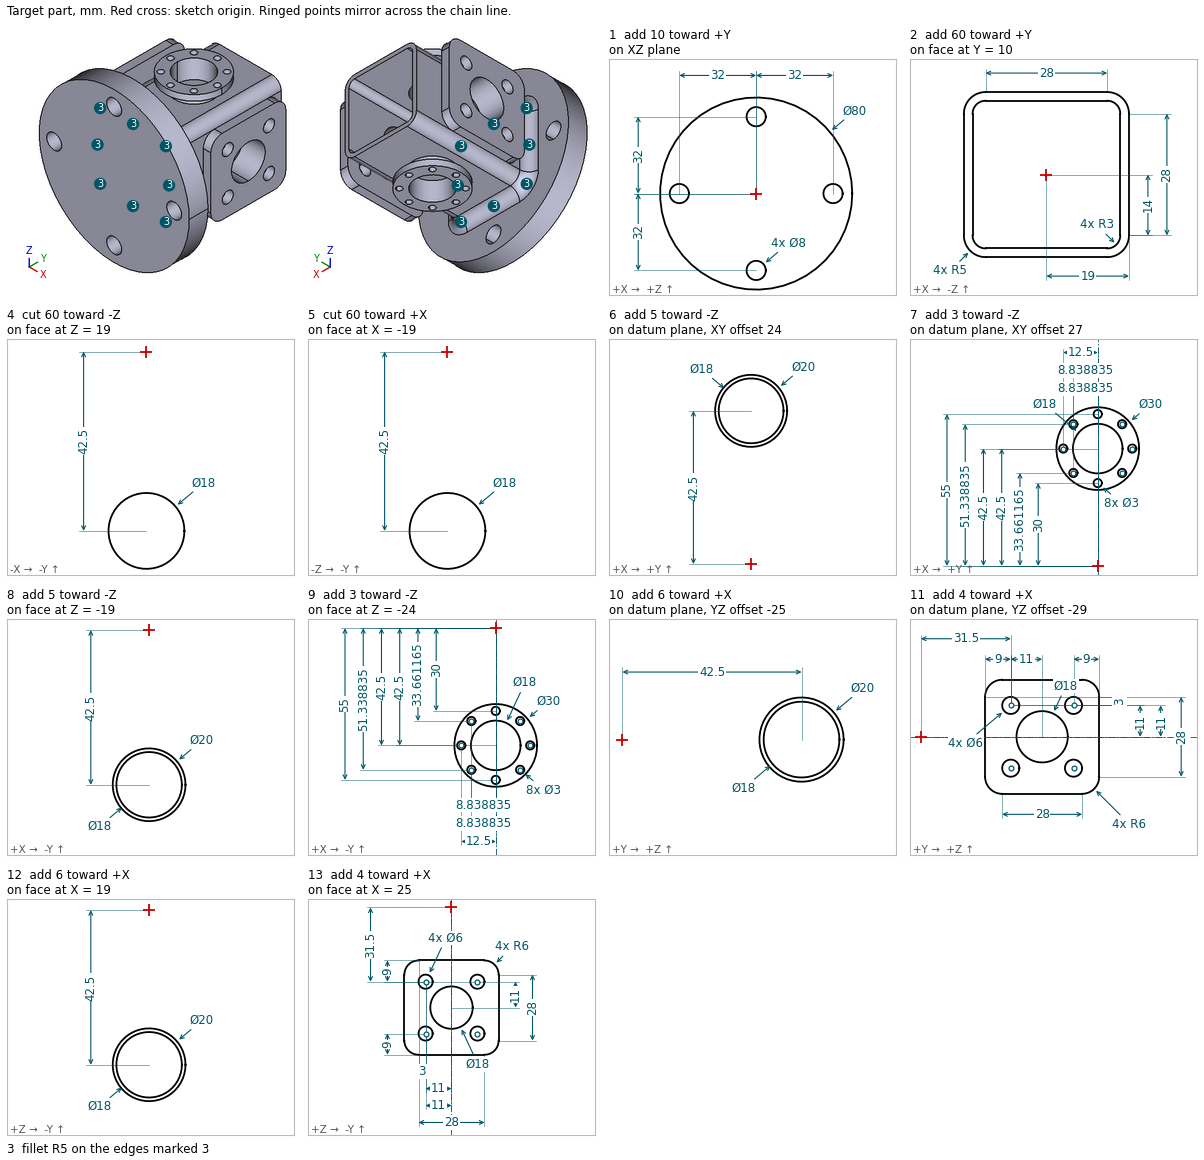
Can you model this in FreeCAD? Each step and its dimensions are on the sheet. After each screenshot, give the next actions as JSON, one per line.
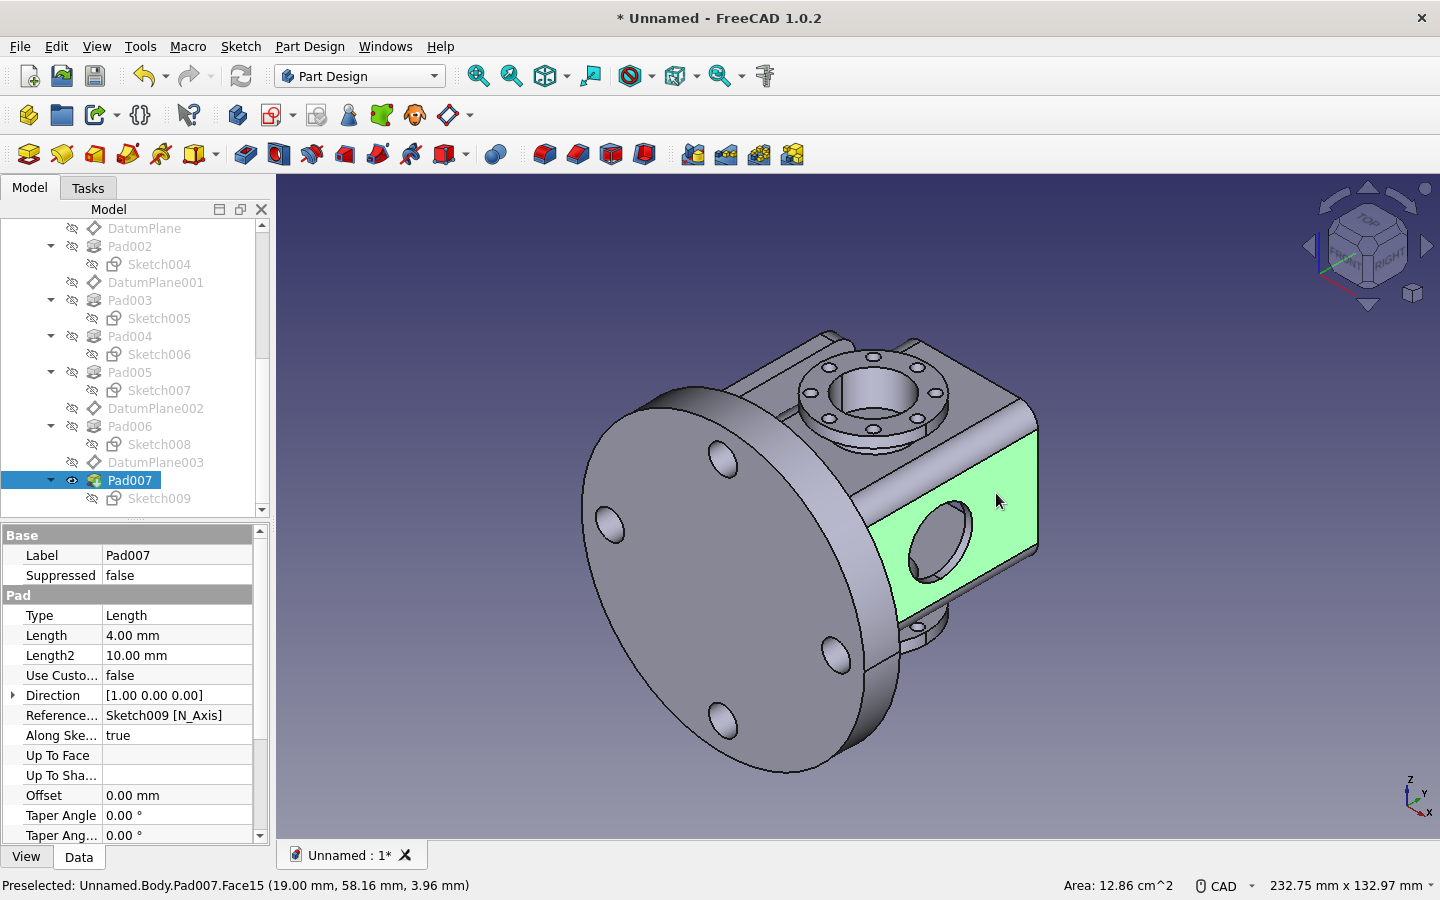
{"action": "left_click", "coordinate": [270, 116]}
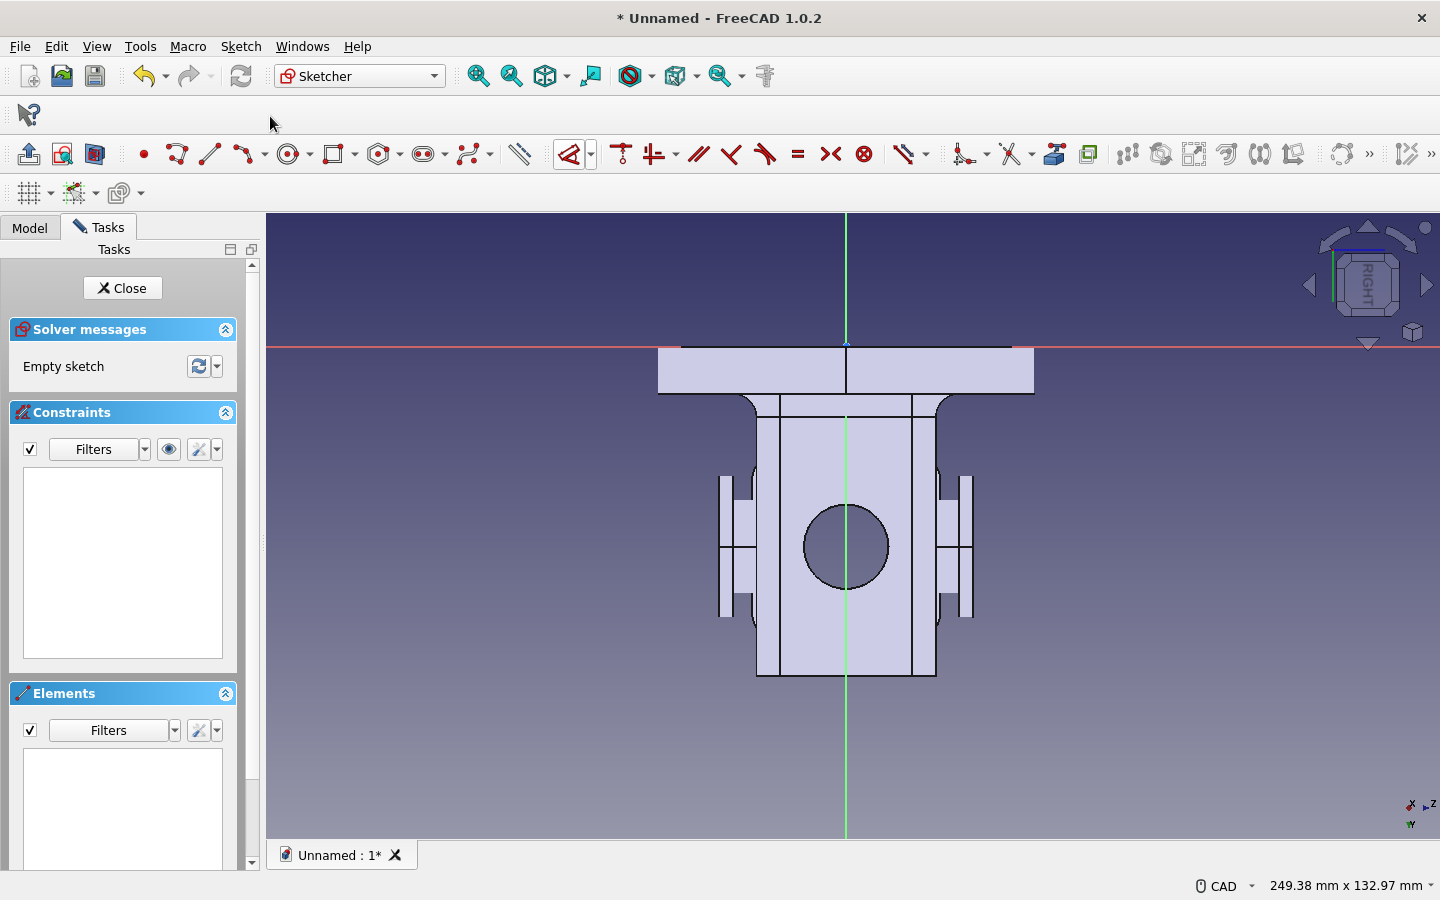
{"action": "scroll", "coordinate": [866, 553], "scroll_direction": "up", "scroll_amount": 7}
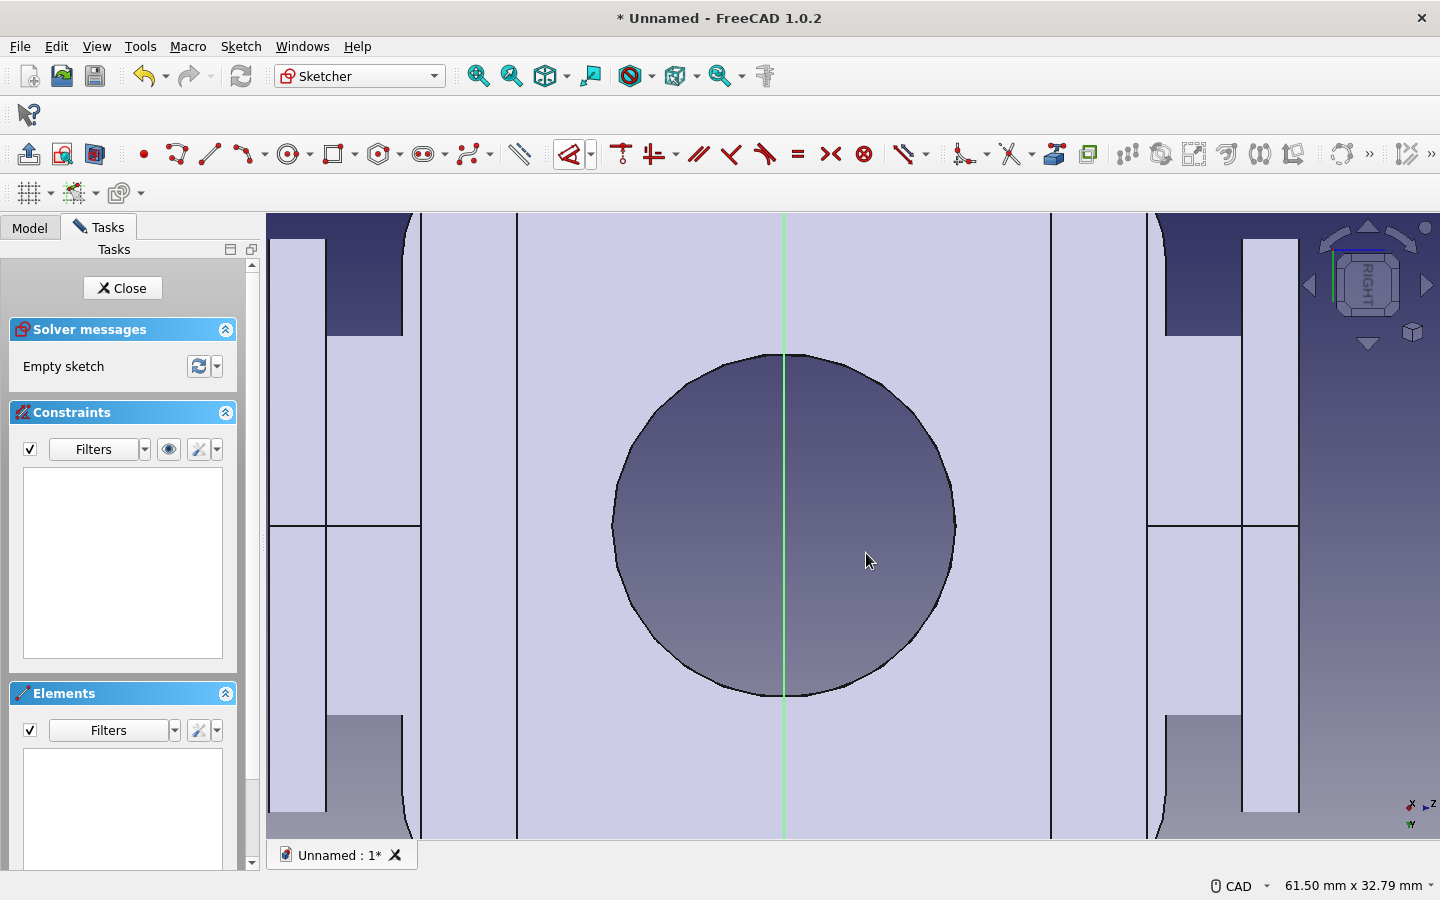
{"action": "key", "text": "g c"}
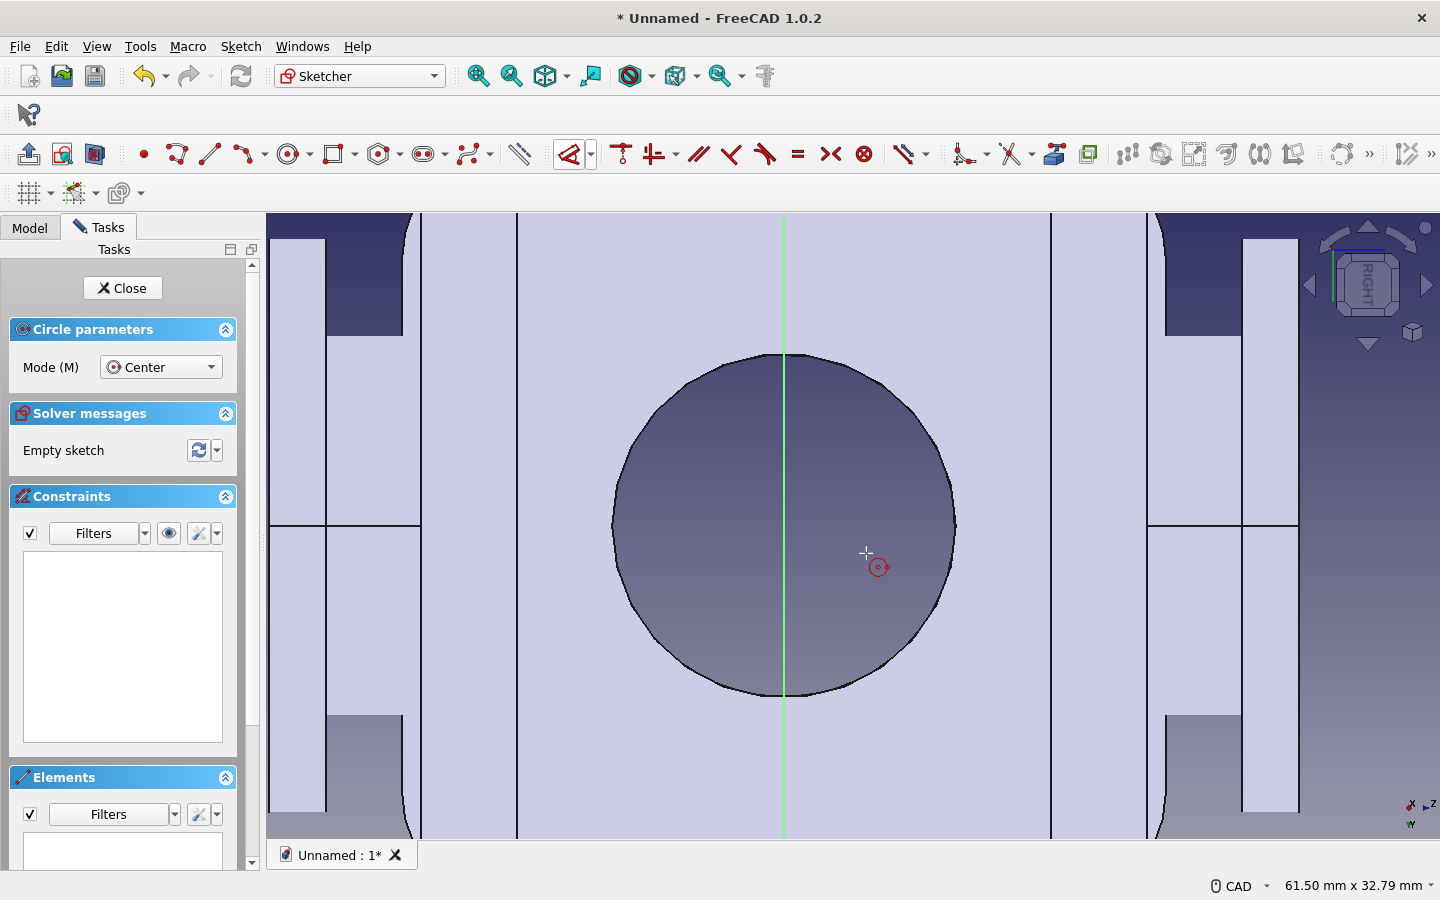
{"action": "left_click", "coordinate": [784, 526]}
{"action": "mouse_move", "coordinate": [919, 391]}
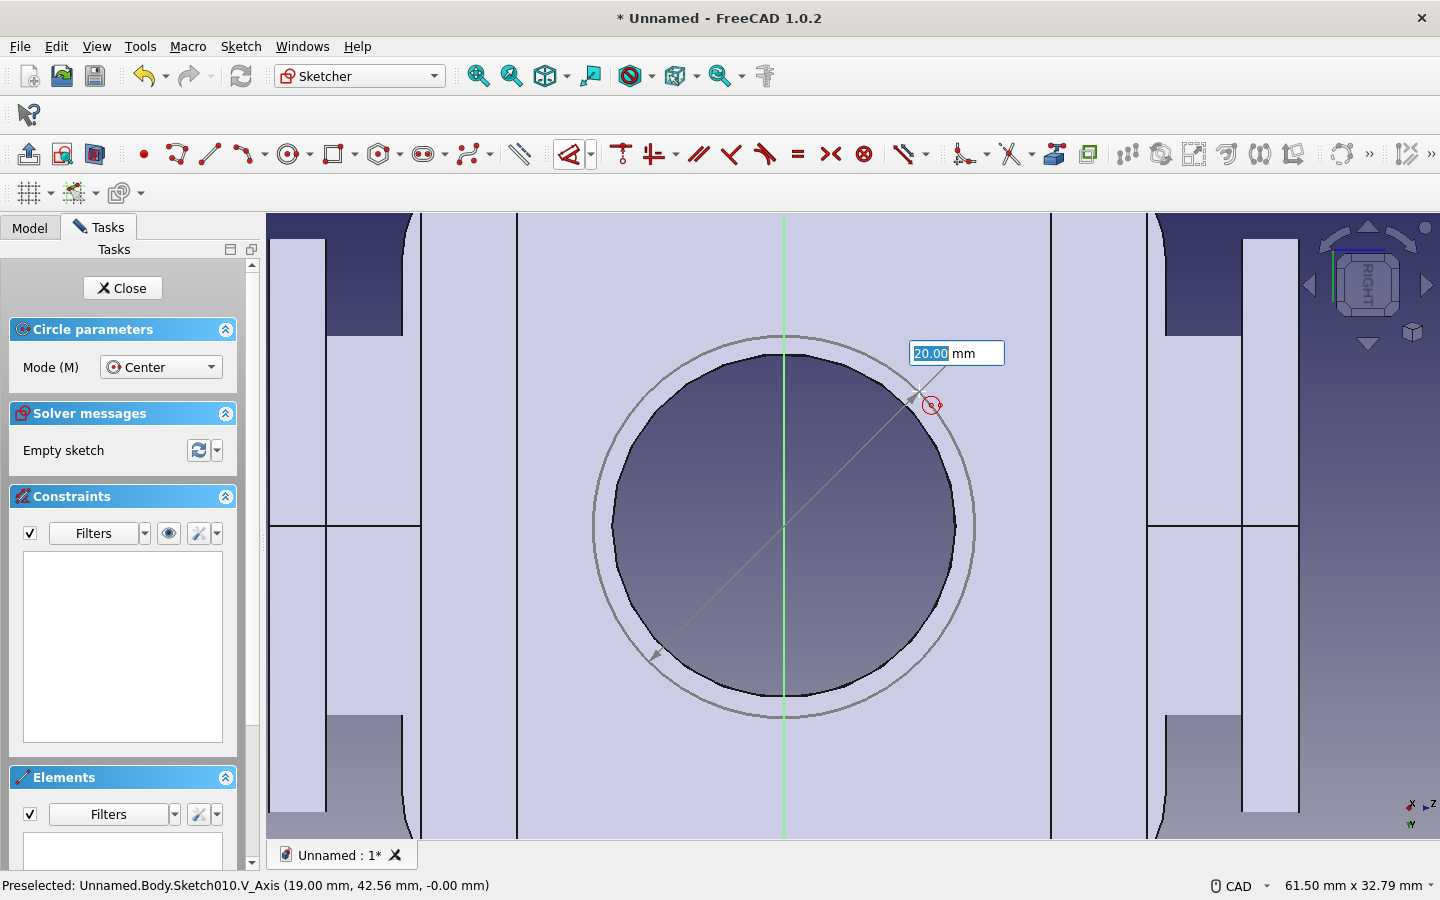
{"action": "type", "text": "20"}
{"action": "key", "text": "Return"}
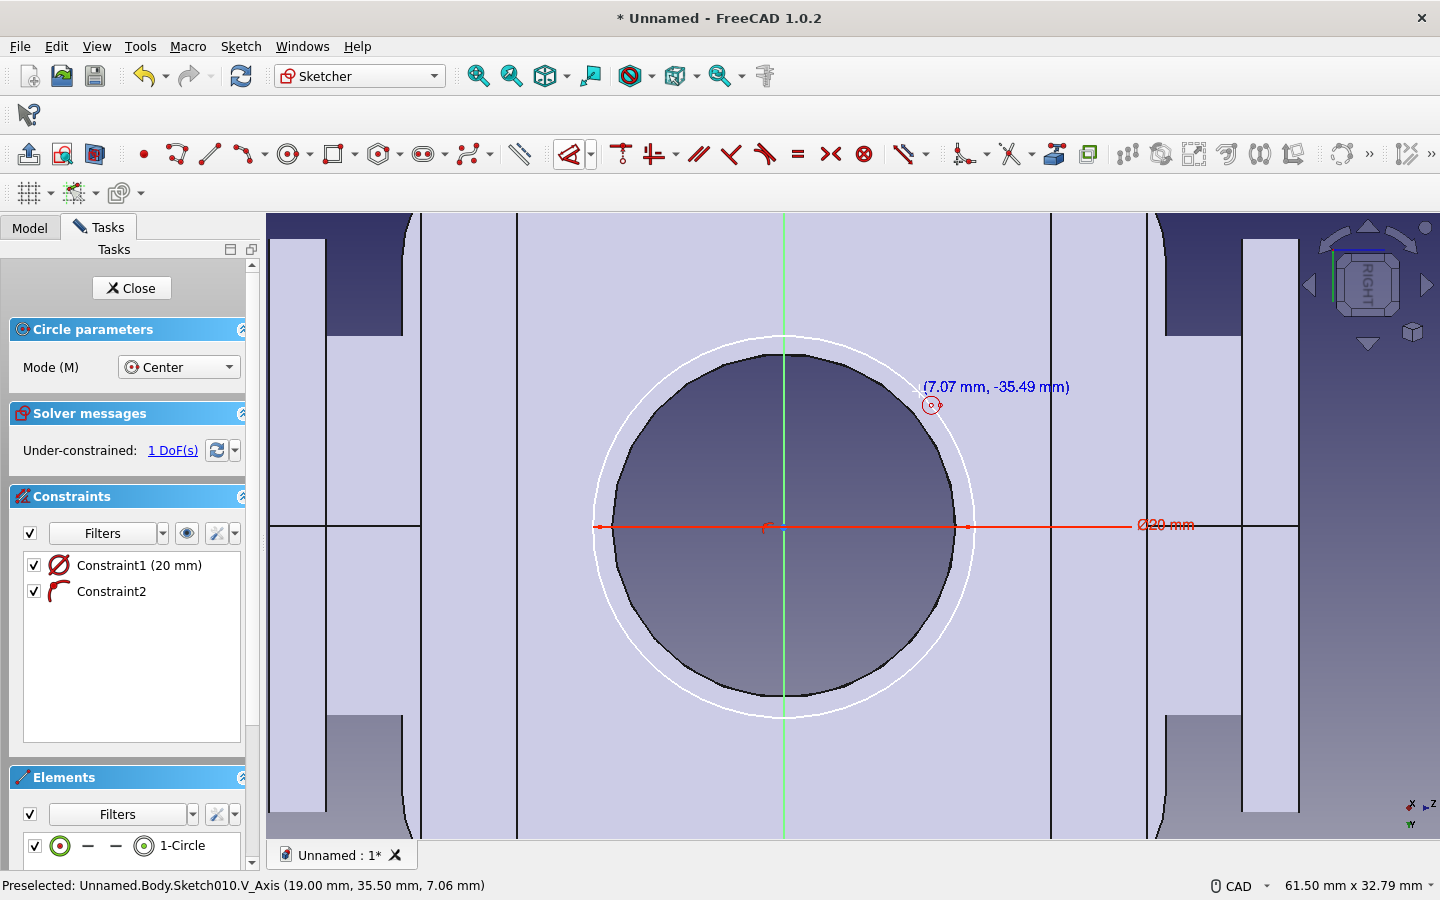
{"action": "left_click", "coordinate": [784, 527]}
{"action": "mouse_move", "coordinate": [905, 404]}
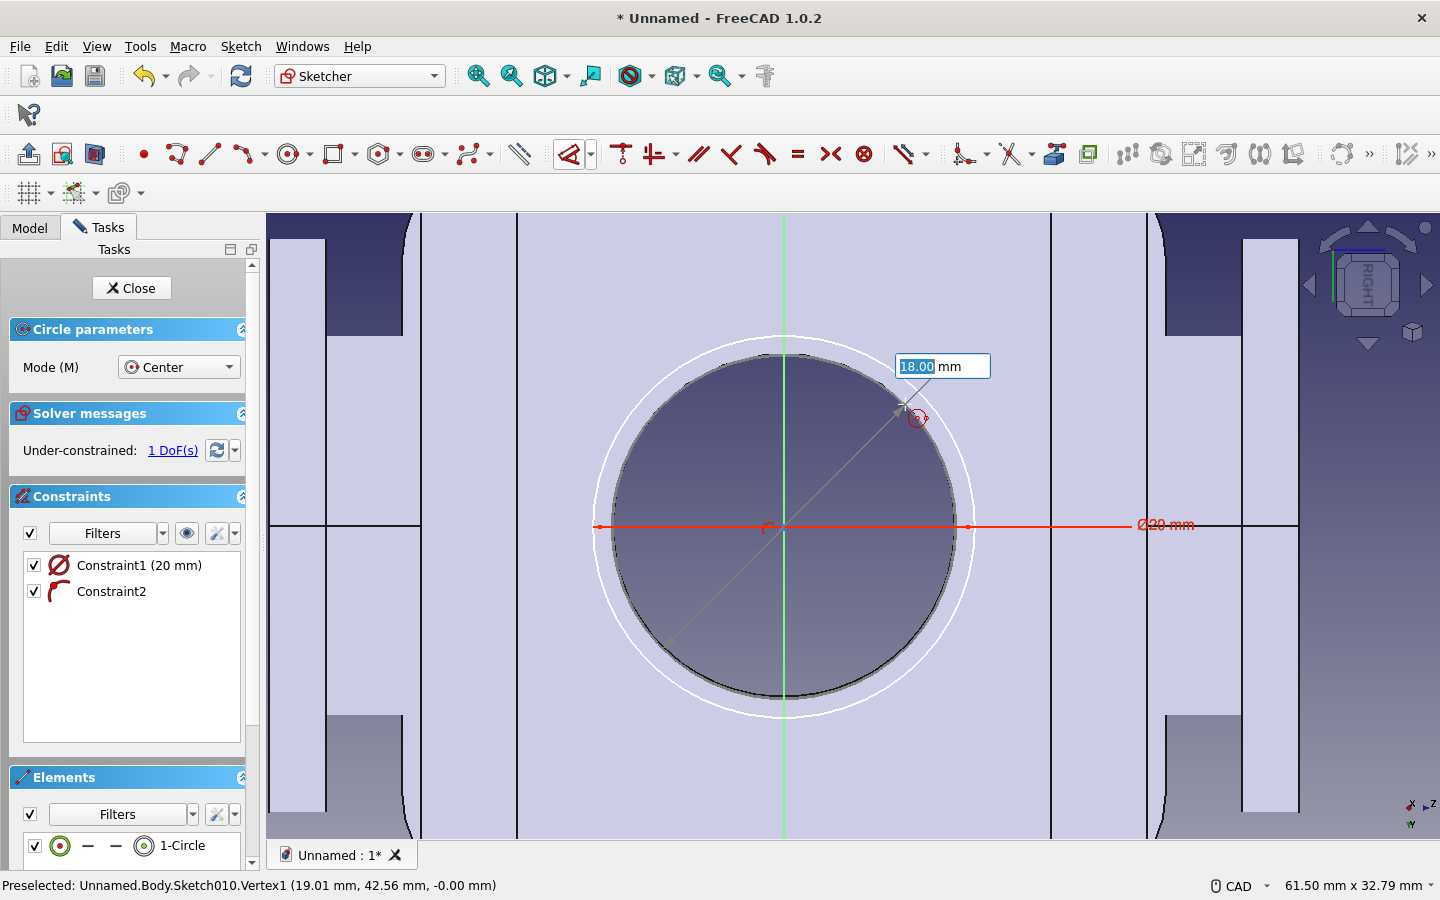
{"action": "type", "text": "18"}
{"action": "key", "text": "Return"}
{"action": "key", "text": "Escape"}